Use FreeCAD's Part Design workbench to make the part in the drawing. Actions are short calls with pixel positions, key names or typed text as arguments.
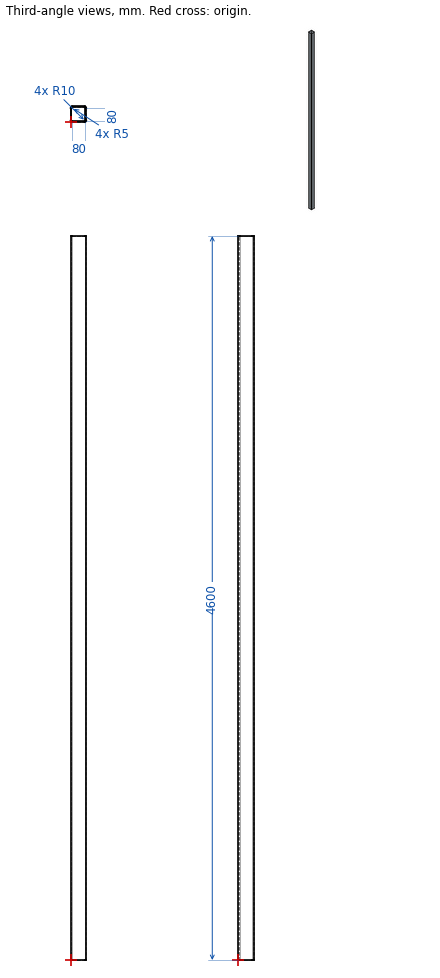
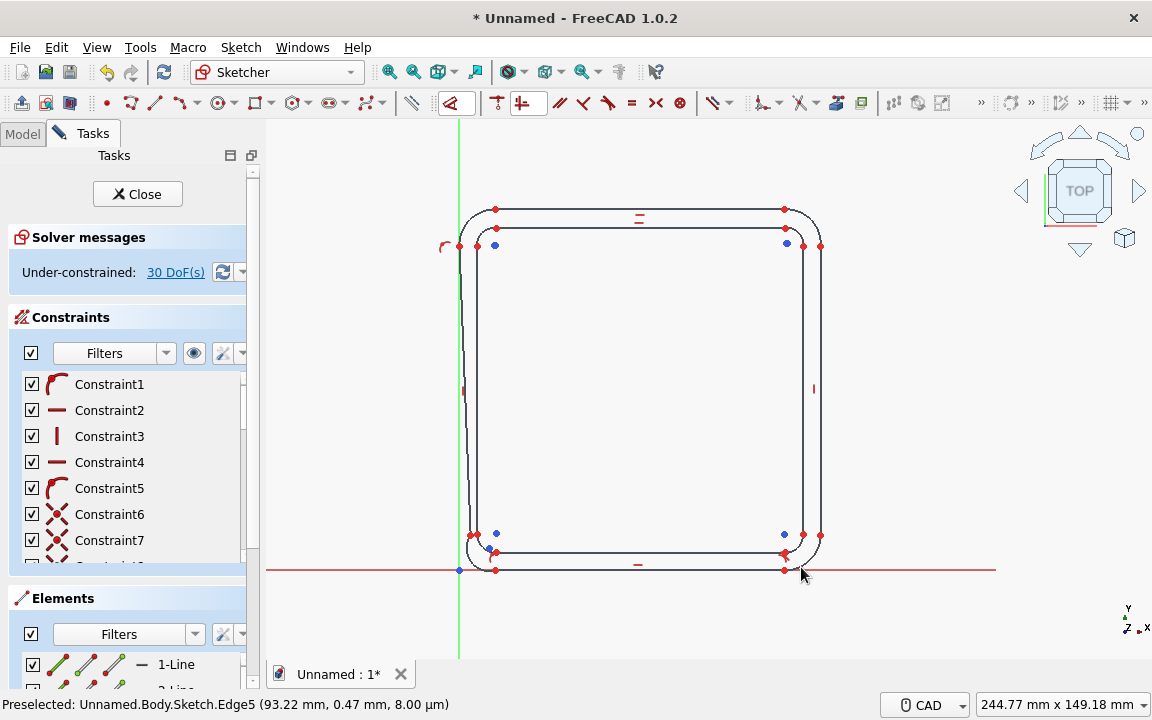
click(582, 570)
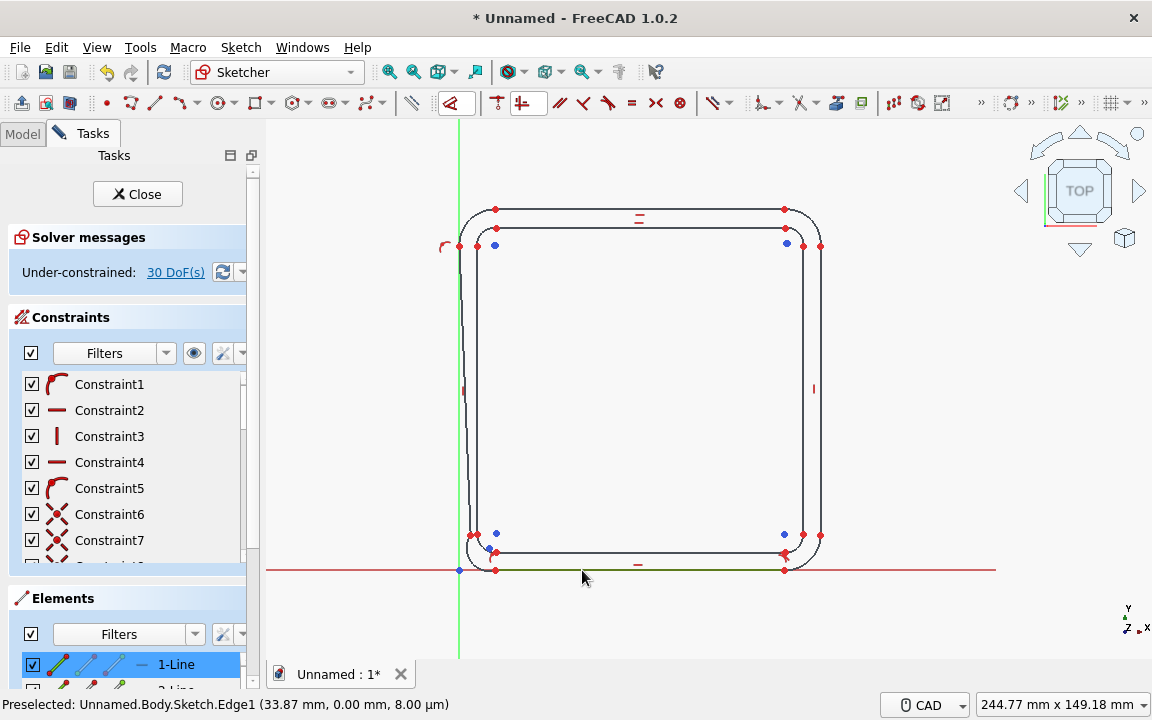
click(479, 569)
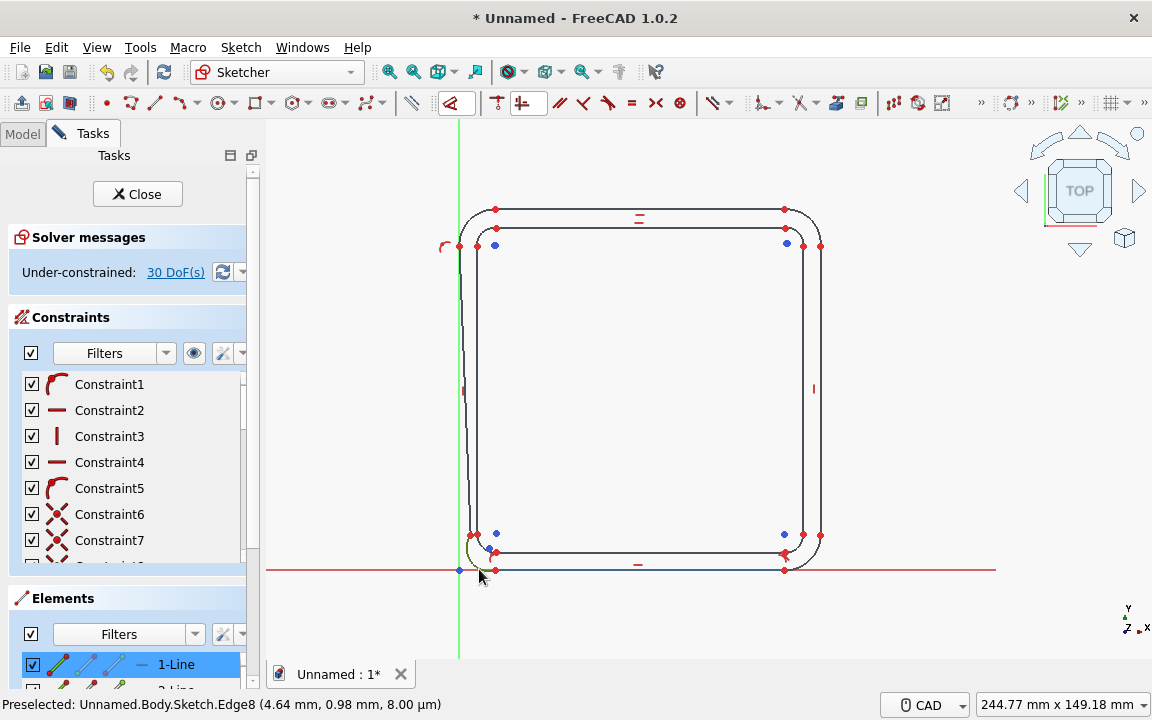
click(608, 104)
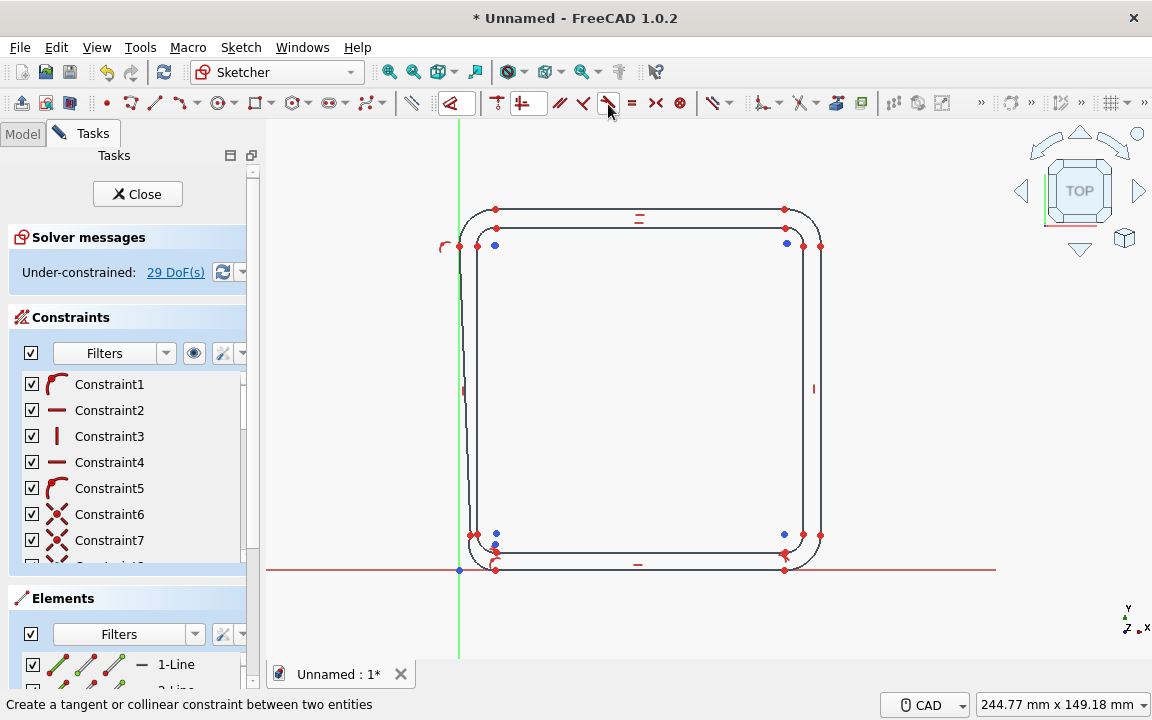
click(821, 449)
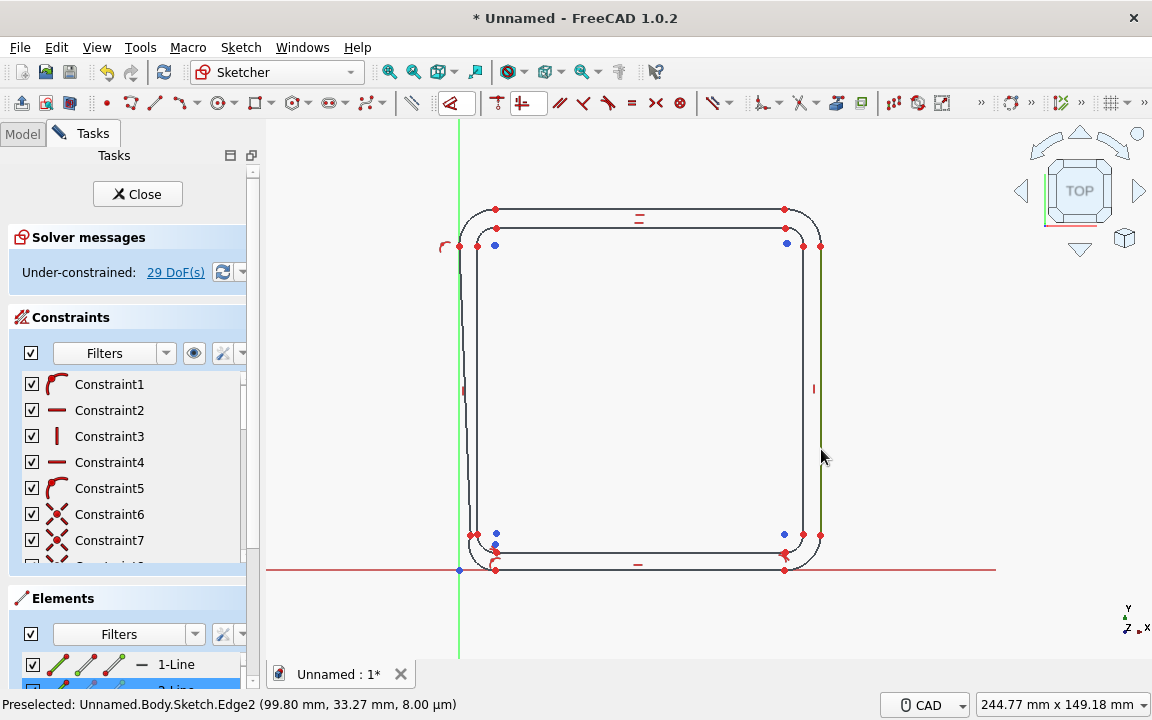
click(801, 567)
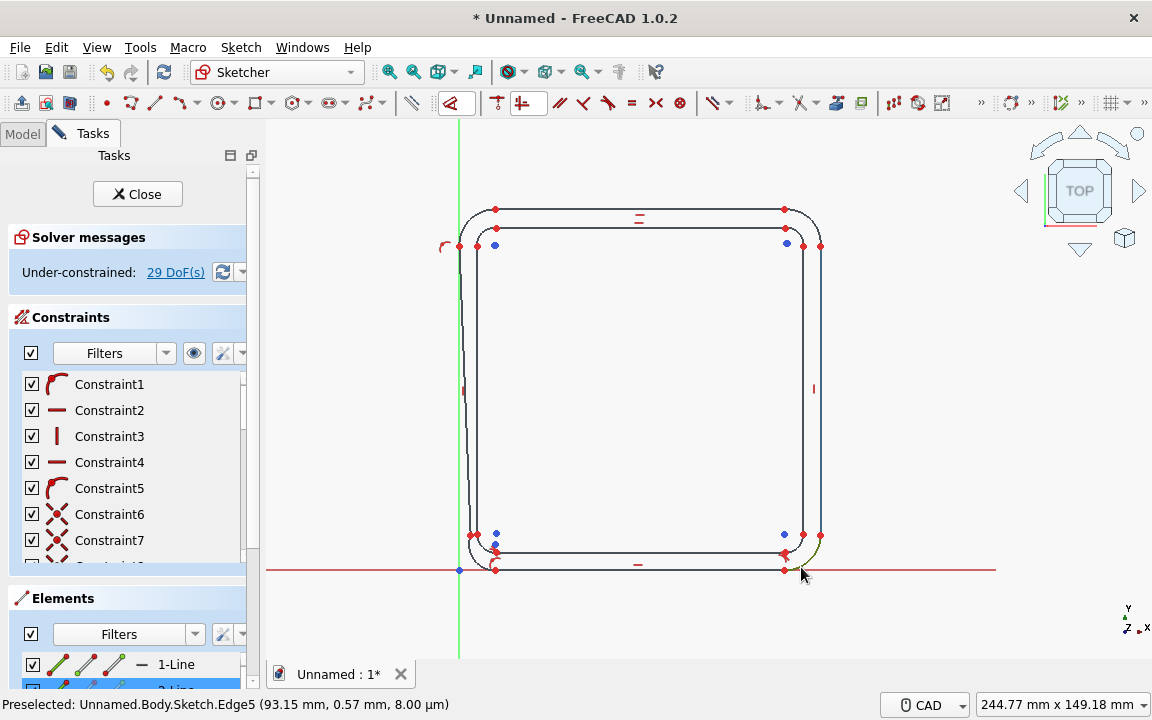
click(608, 104)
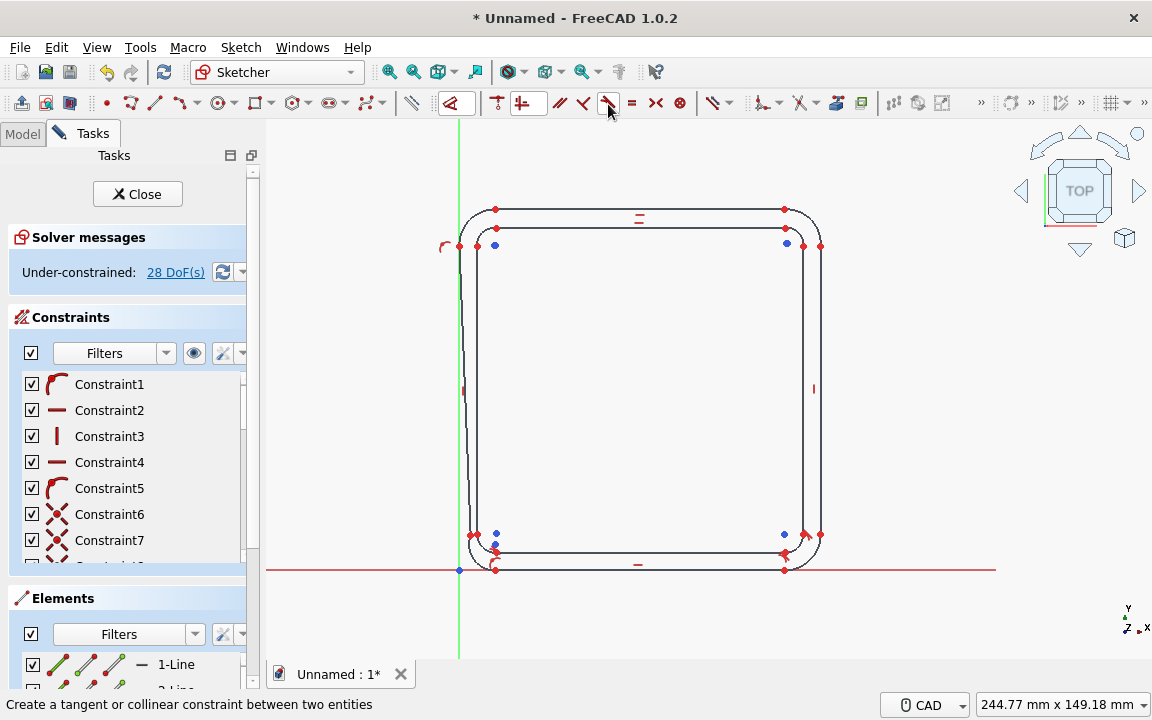
click(821, 448)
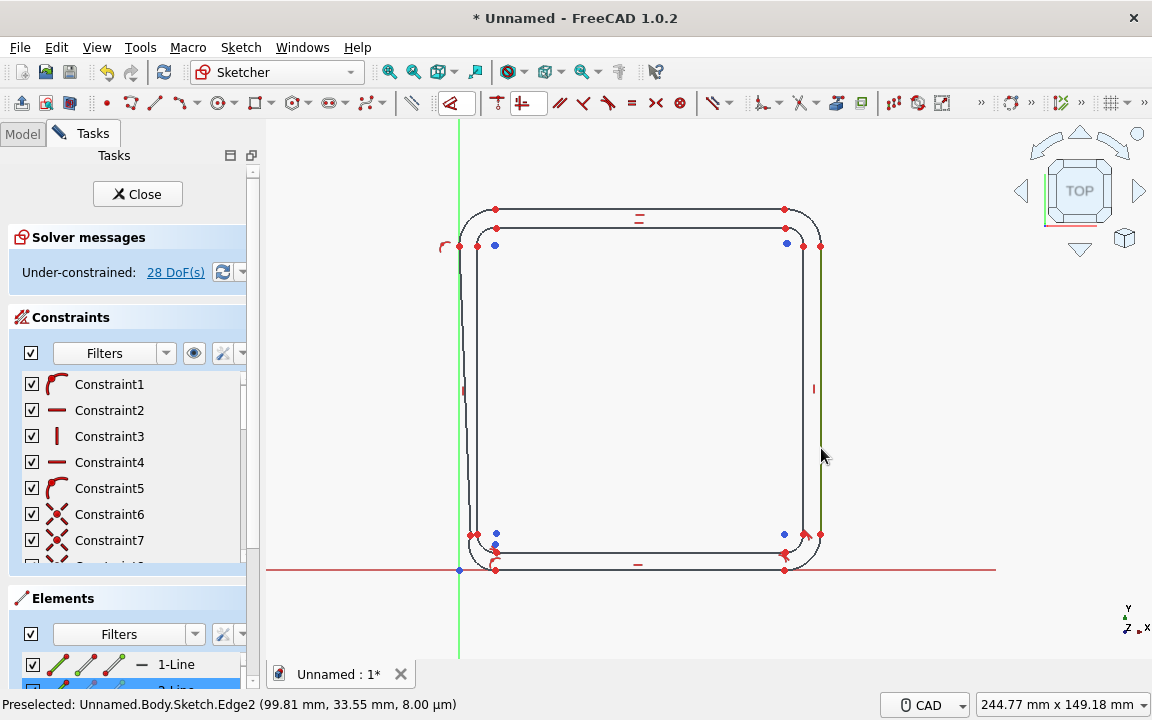
click(817, 229)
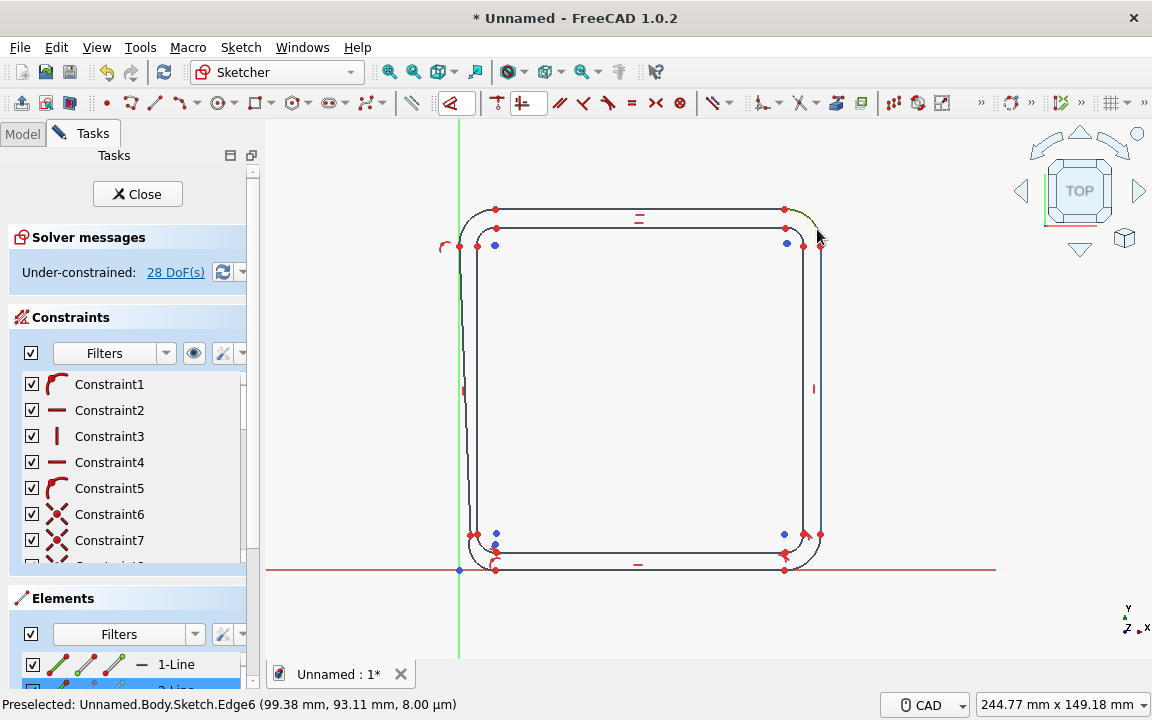
click(608, 104)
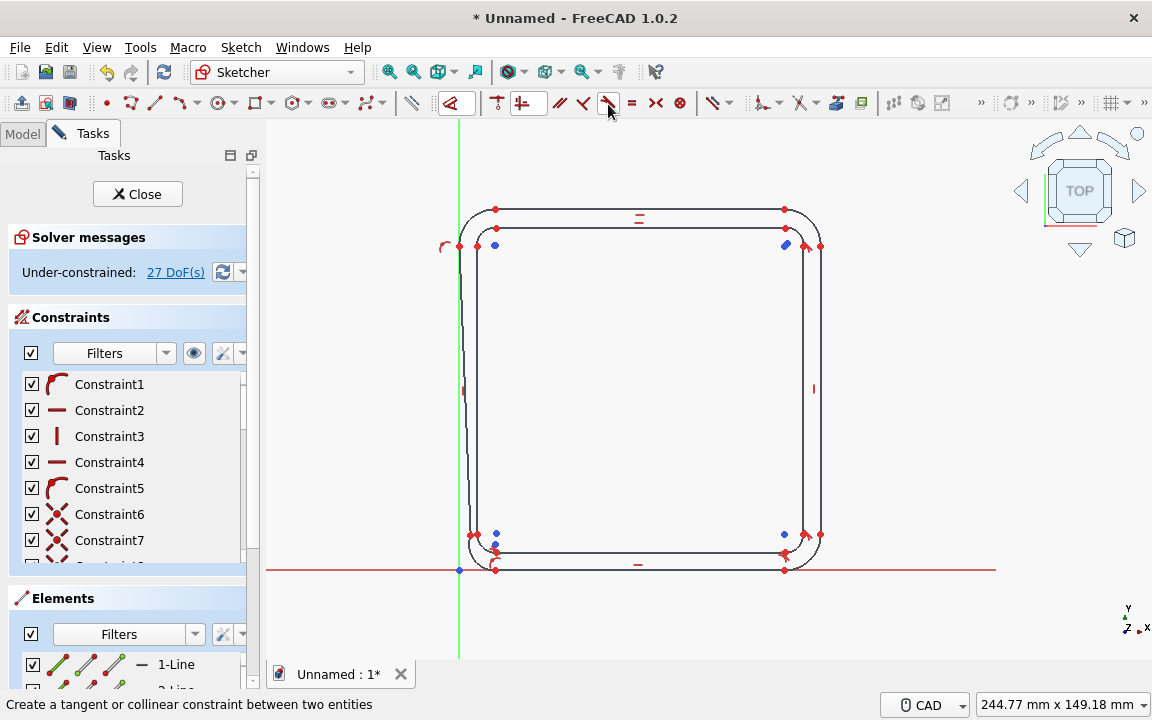
click(698, 209)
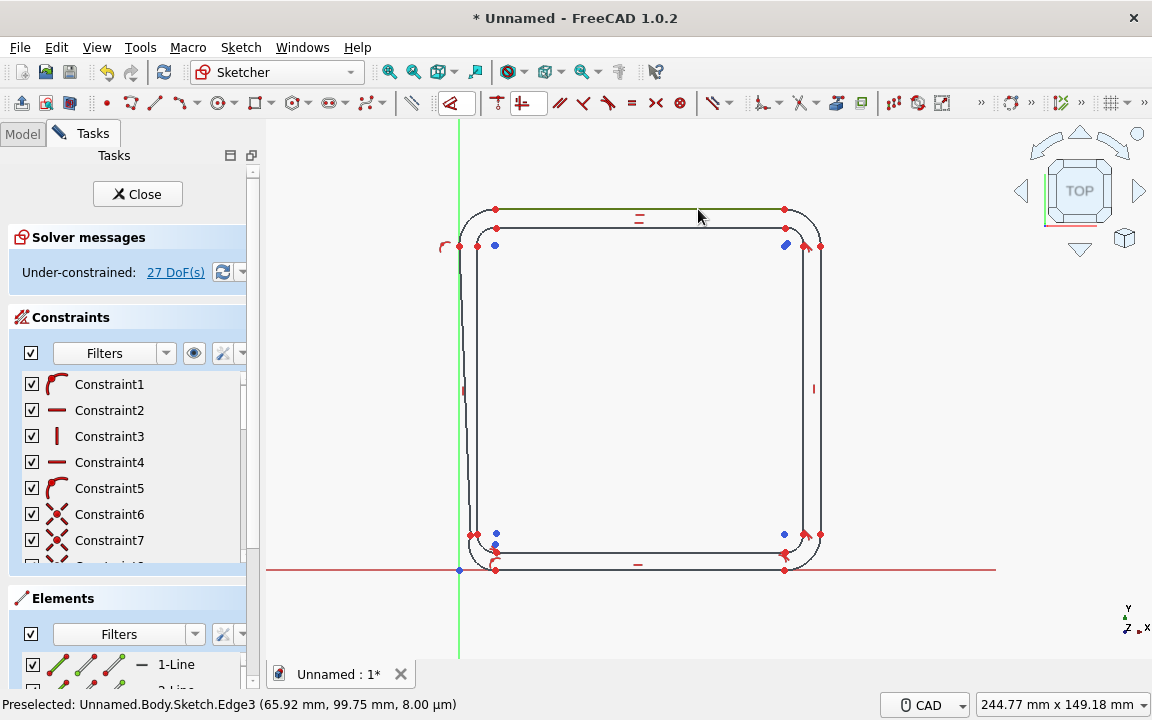
click(817, 229)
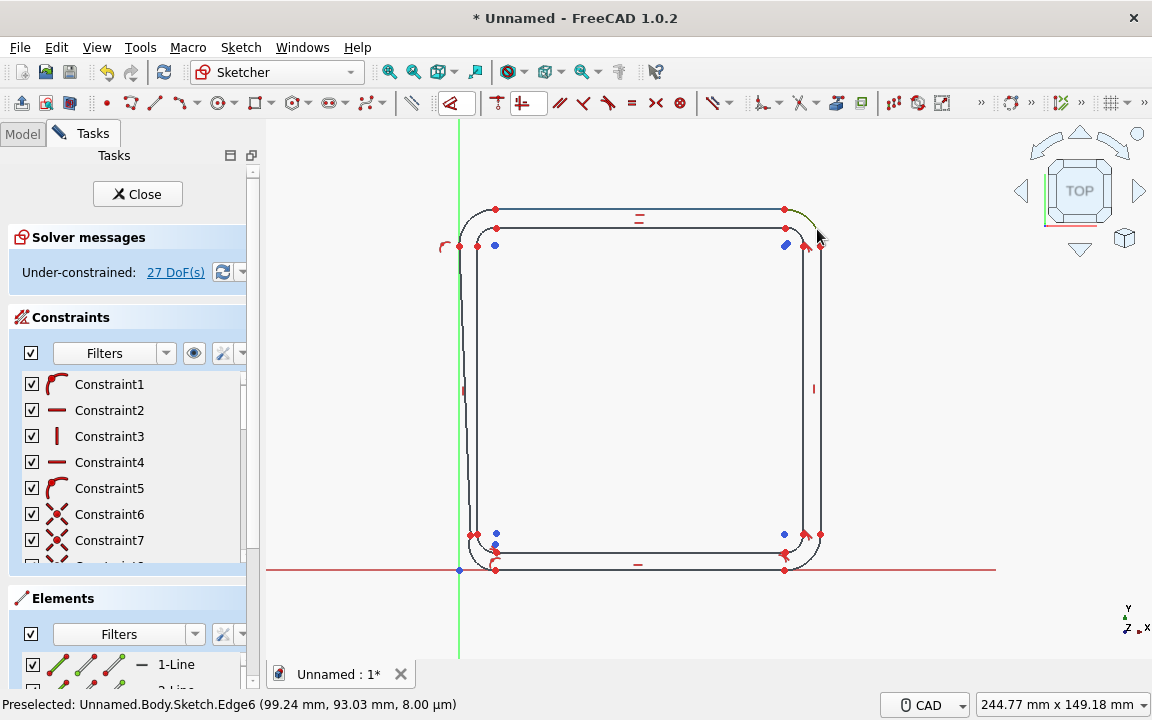
key(t)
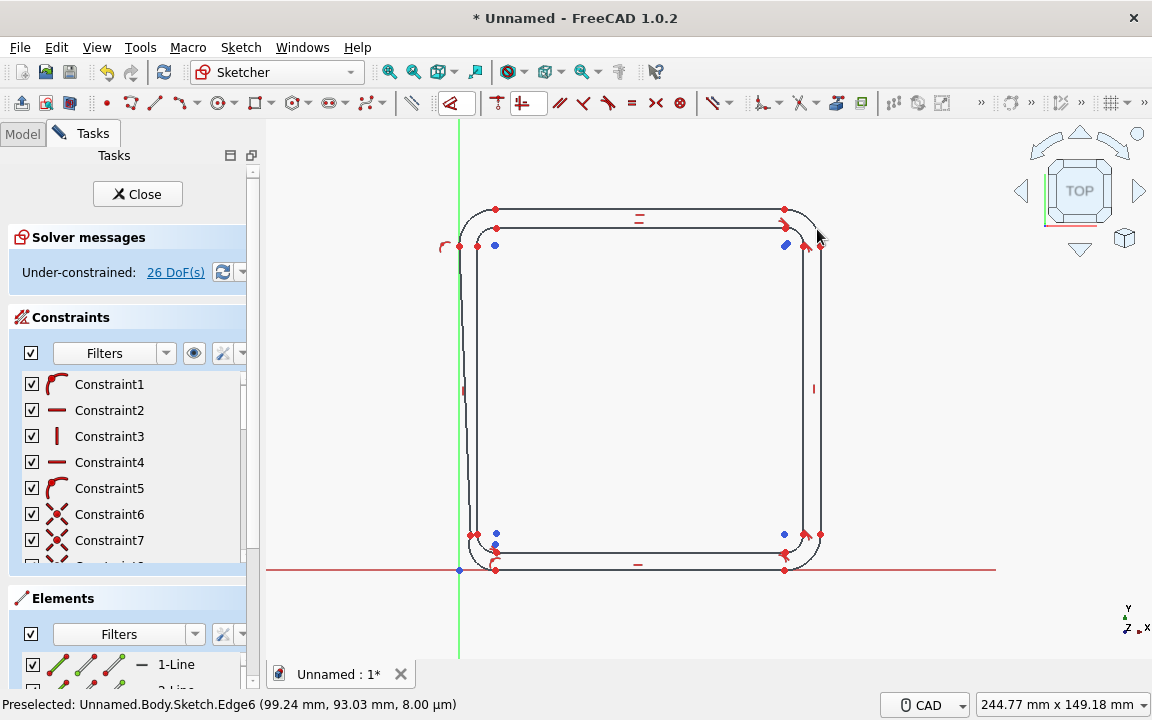
click(697, 209)